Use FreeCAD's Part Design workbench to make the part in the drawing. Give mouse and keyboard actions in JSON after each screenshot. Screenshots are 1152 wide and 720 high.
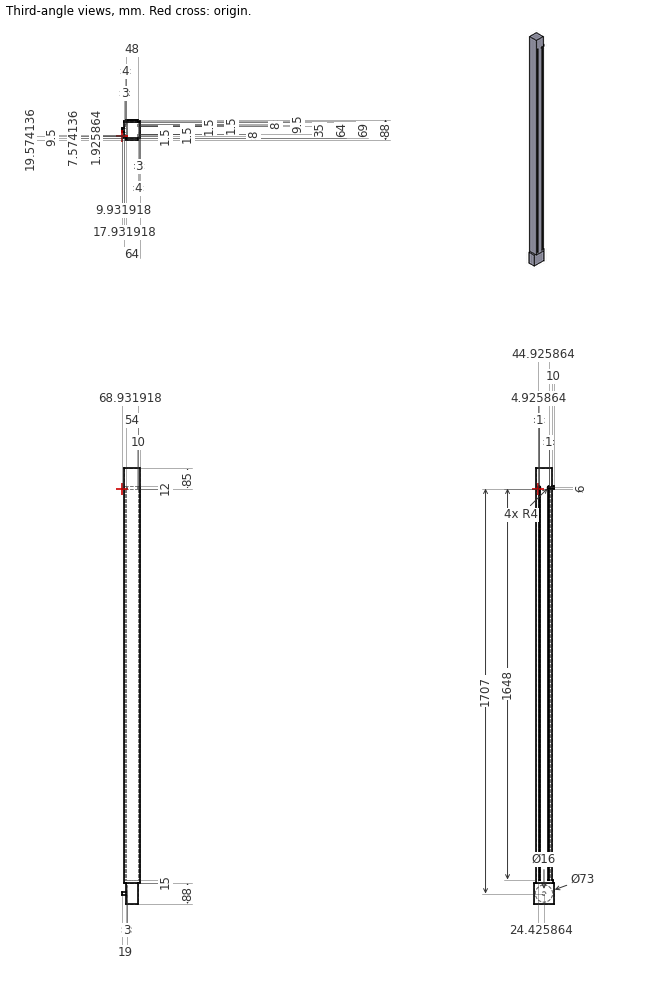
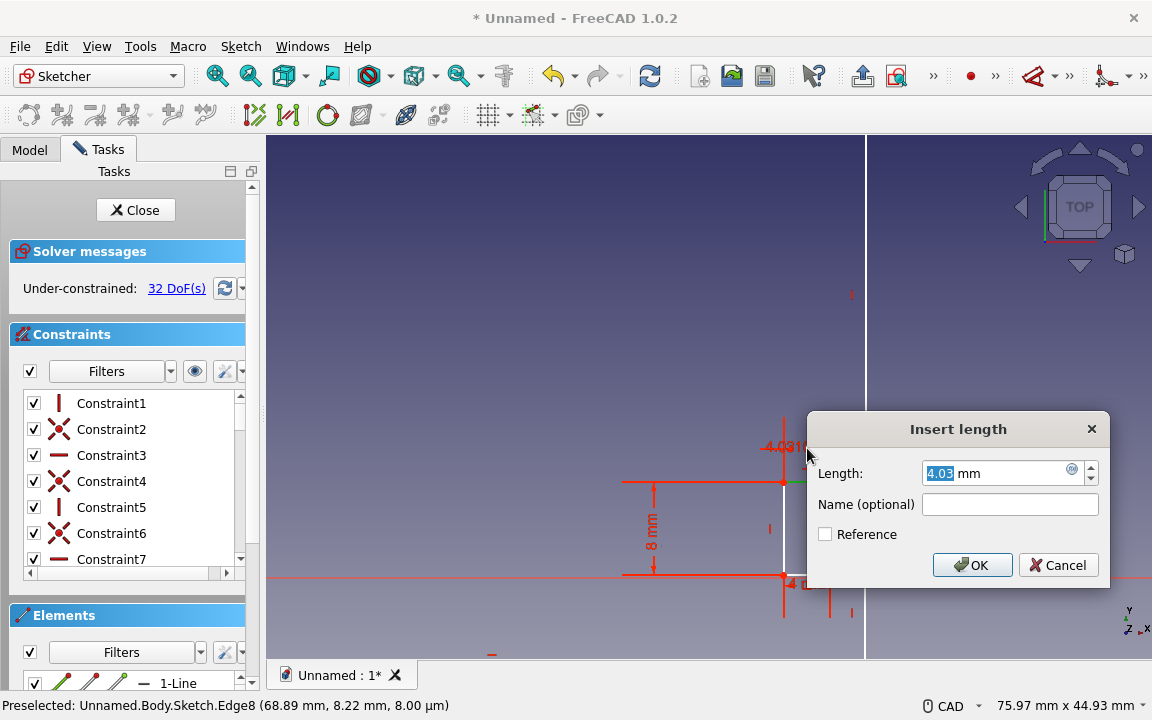
{"action": "type", "text": "4"}
{"action": "key", "text": "Return"}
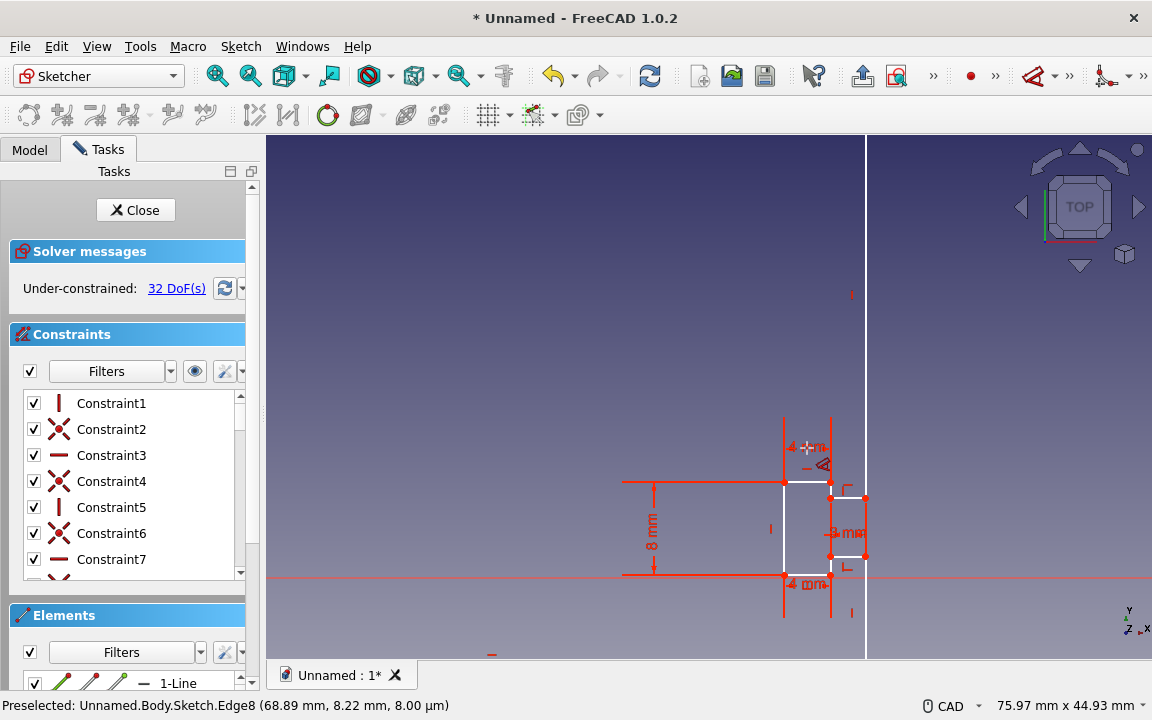
{"action": "scroll", "coordinate": [841, 498], "scroll_direction": "up", "scroll_amount": 2}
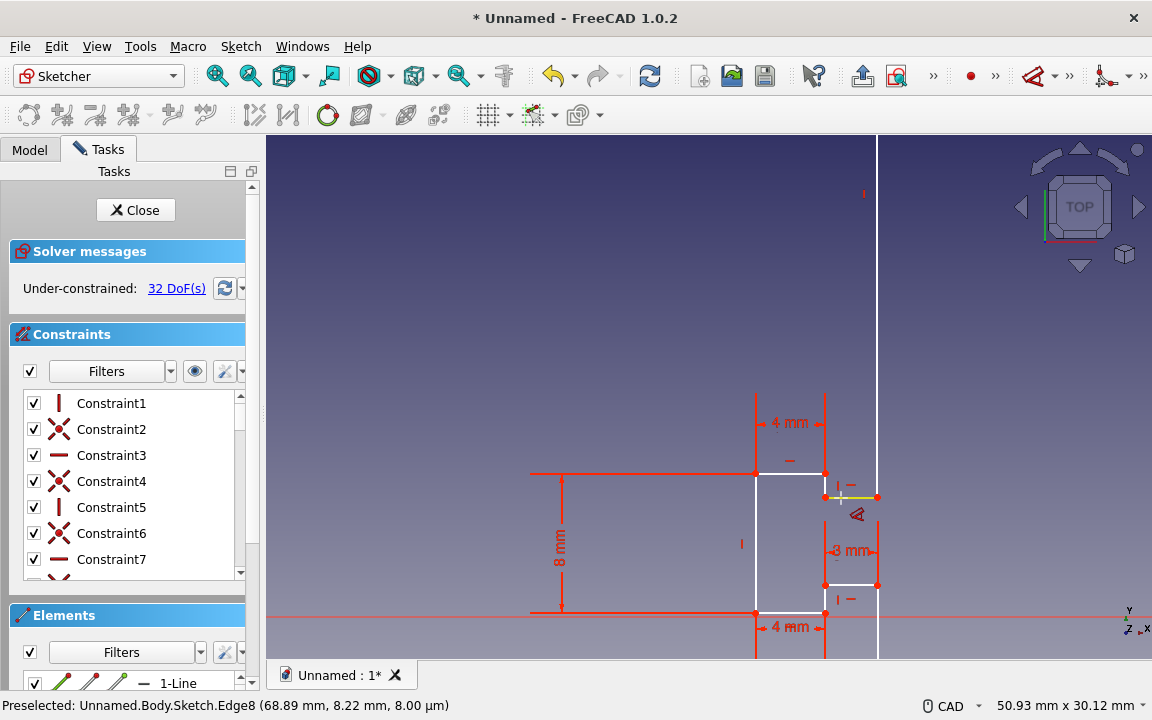
{"action": "left_click", "coordinate": [841, 498]}
{"action": "left_click", "coordinate": [851, 464]}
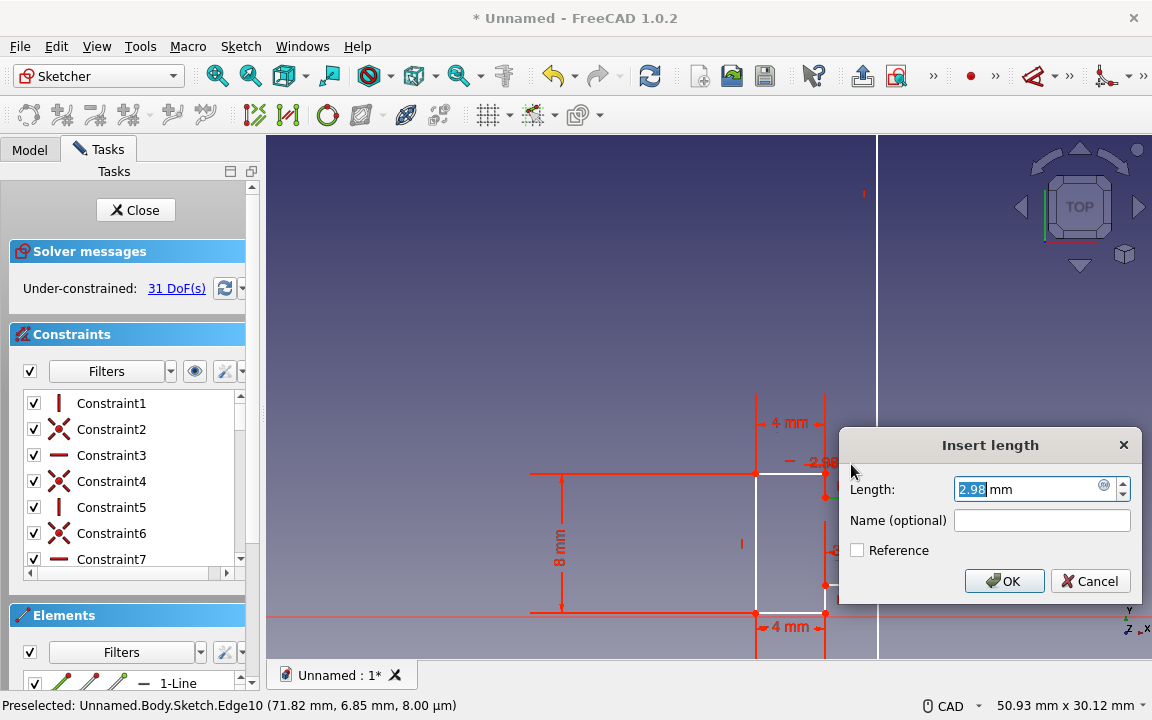
{"action": "type", "text": "3"}
{"action": "key", "text": "Return"}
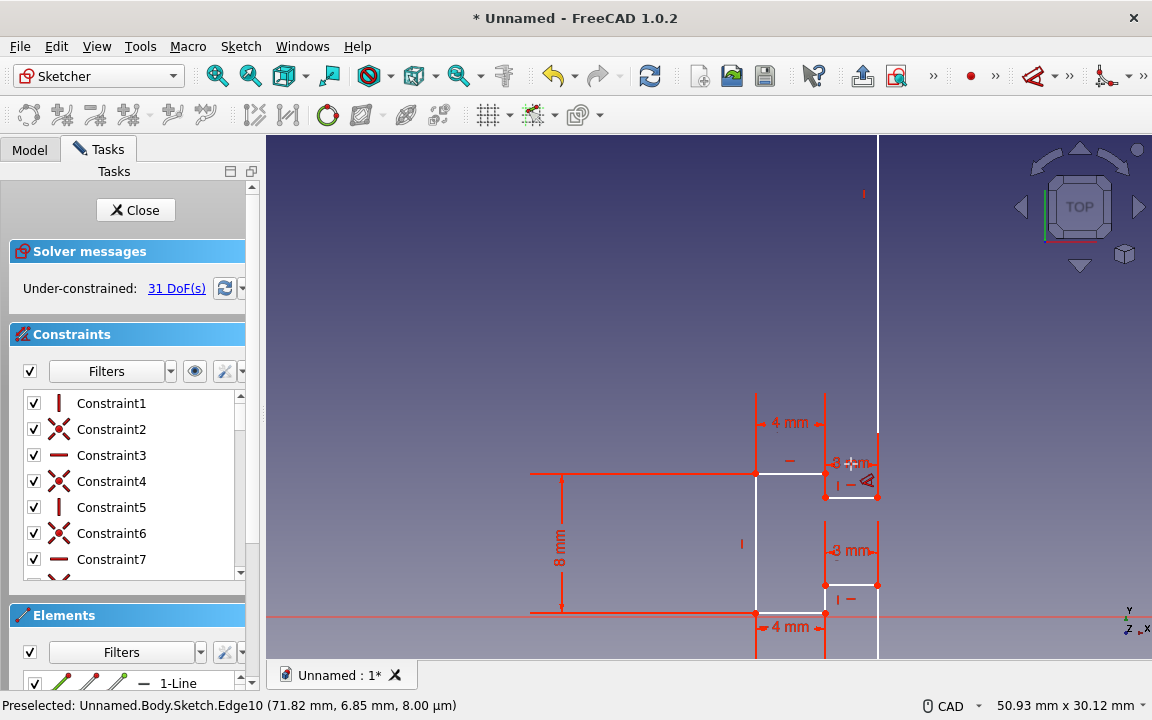
{"action": "scroll", "coordinate": [815, 485], "scroll_direction": "down", "scroll_amount": 6}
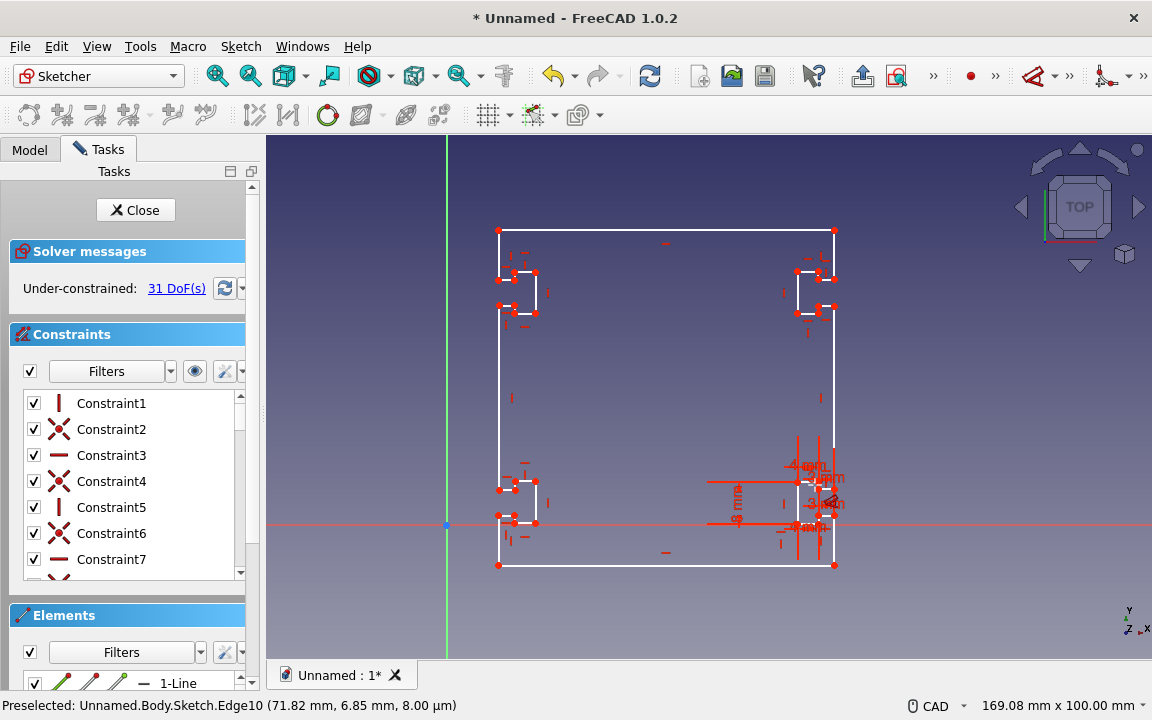
{"action": "scroll", "coordinate": [830, 306], "scroll_direction": "up", "scroll_amount": 6}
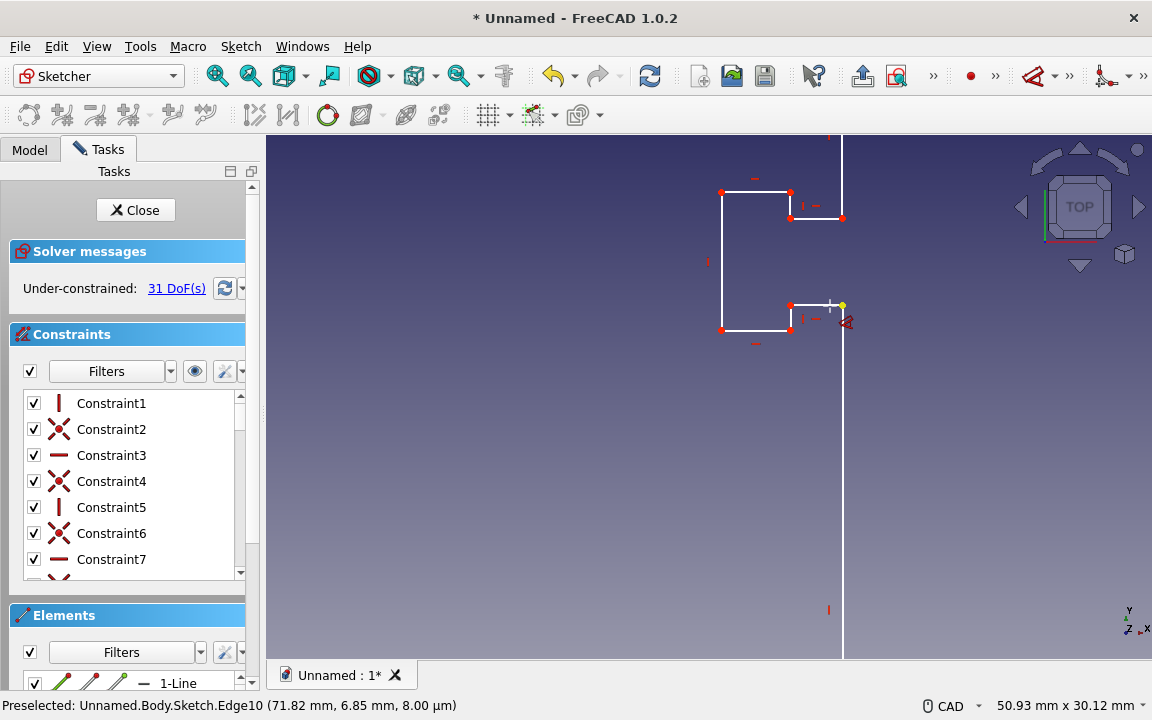
{"action": "left_click", "coordinate": [827, 305]}
{"action": "left_click", "coordinate": [817, 271]}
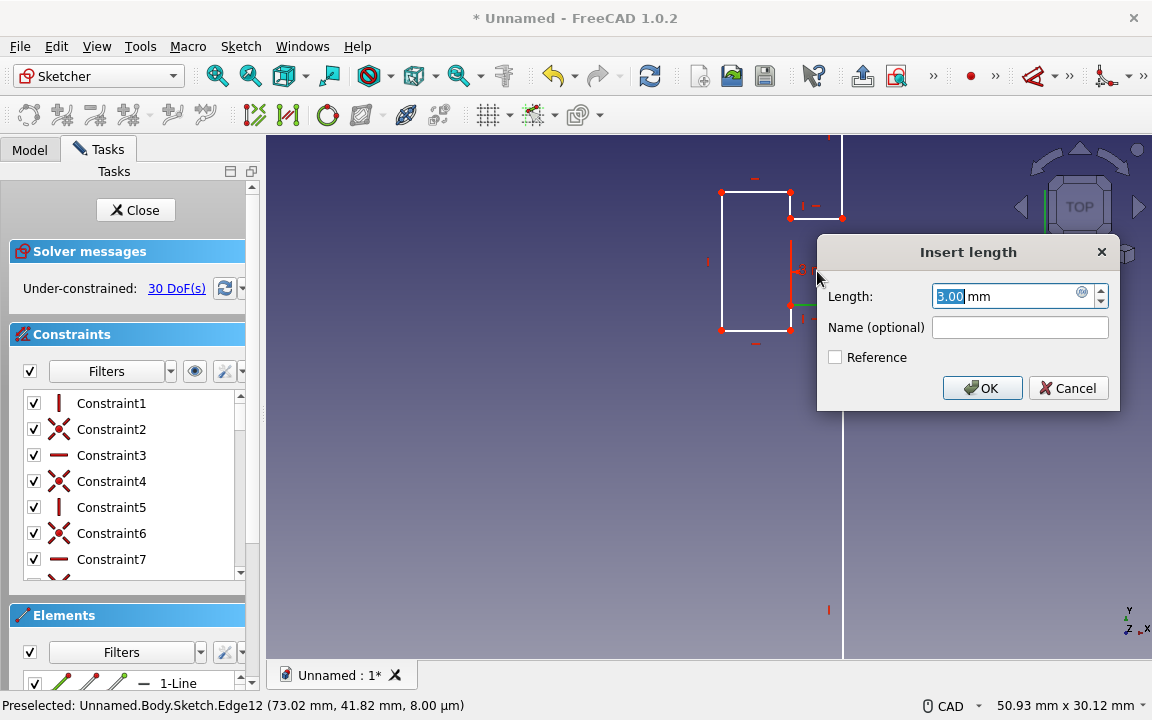
{"action": "type", "text": "3"}
{"action": "key", "text": "Return"}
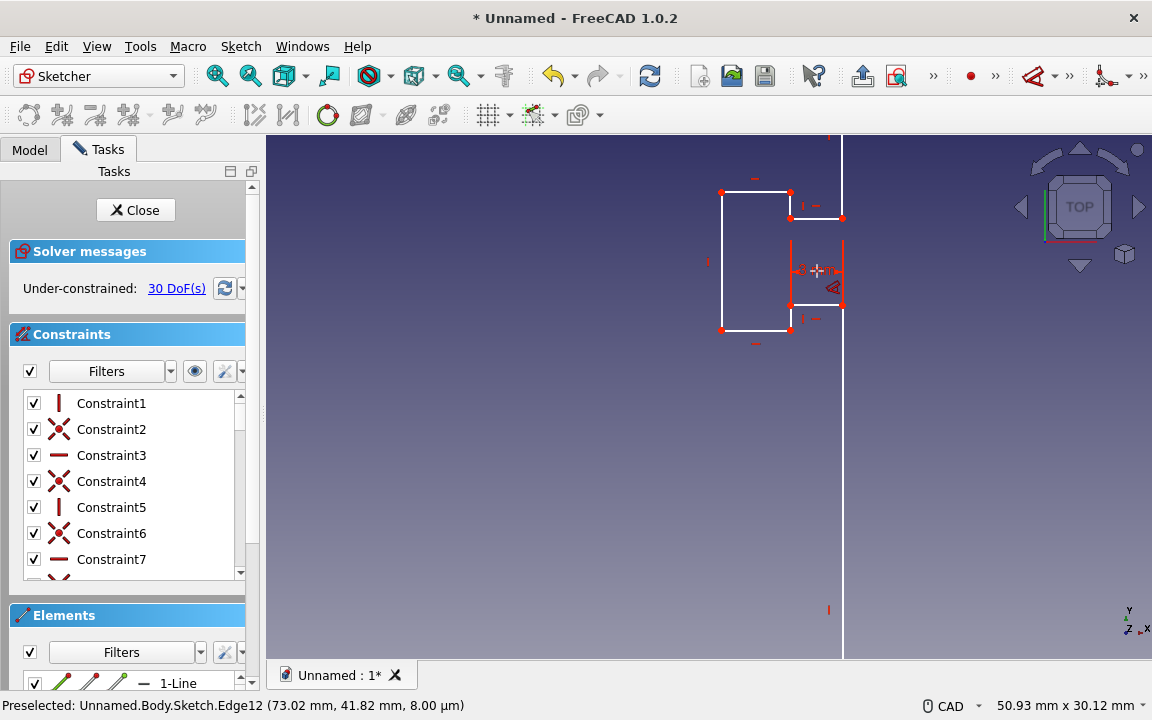
{"action": "left_click", "coordinate": [770, 331]}
{"action": "left_click", "coordinate": [756, 297]}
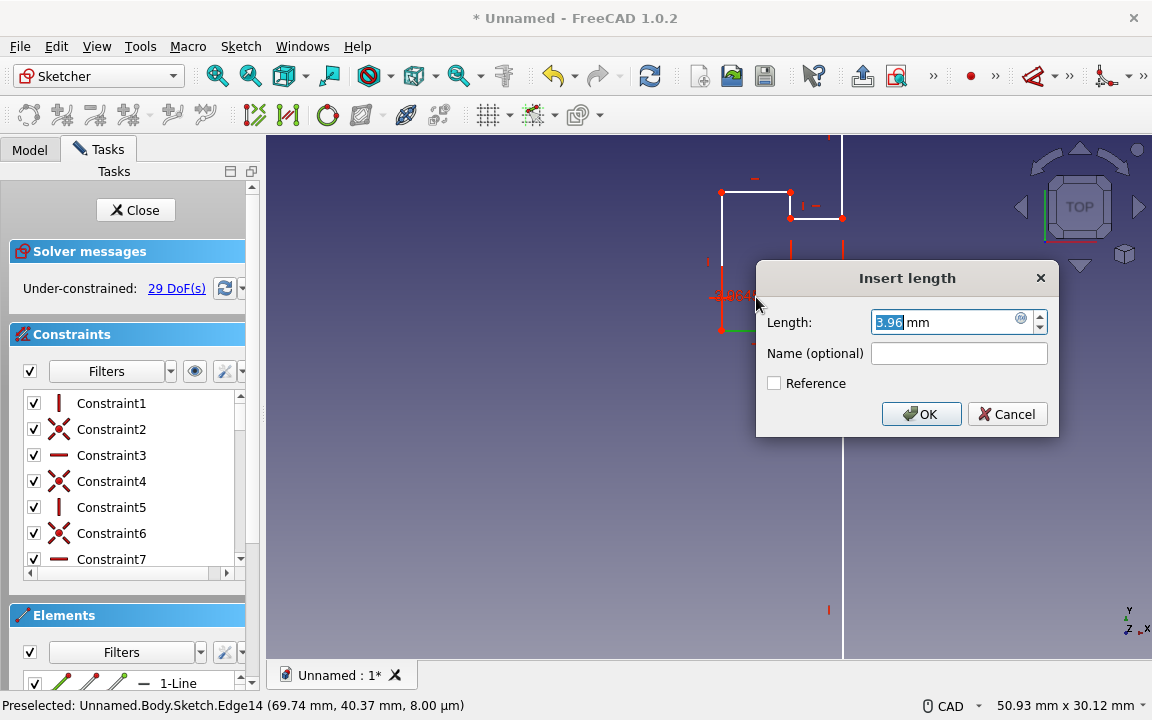
{"action": "type", "text": "4"}
{"action": "key", "text": "Return"}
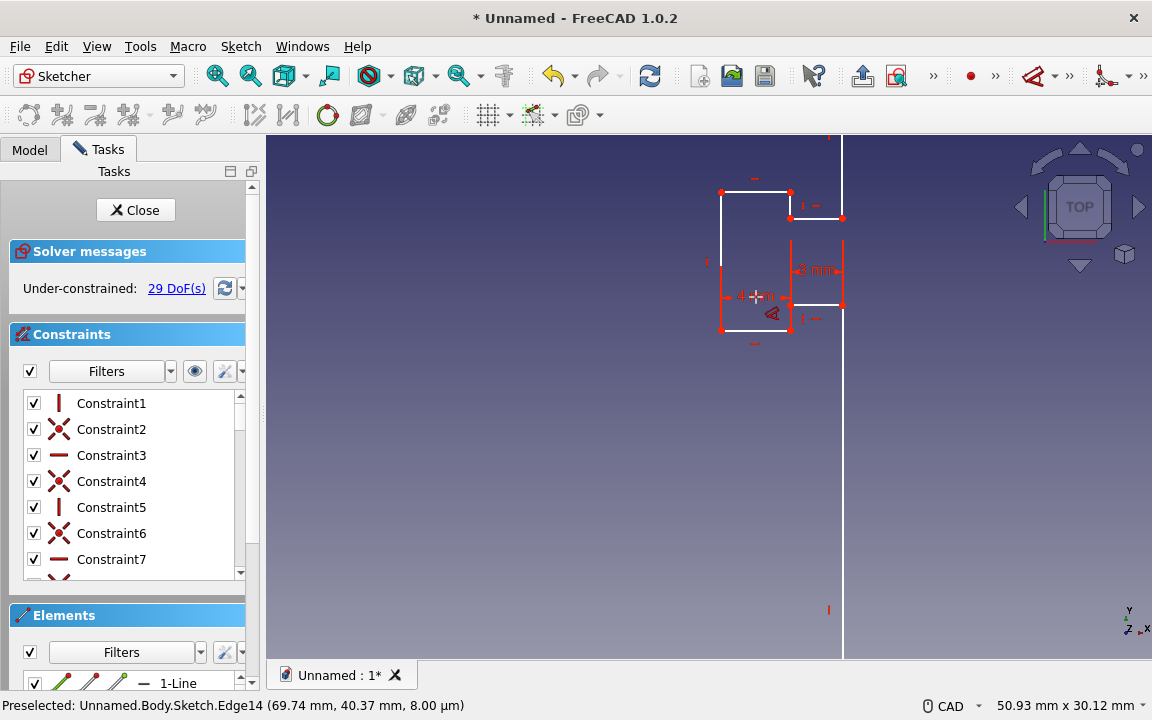
{"action": "scroll", "coordinate": [830, 306], "scroll_direction": "down", "scroll_amount": 6}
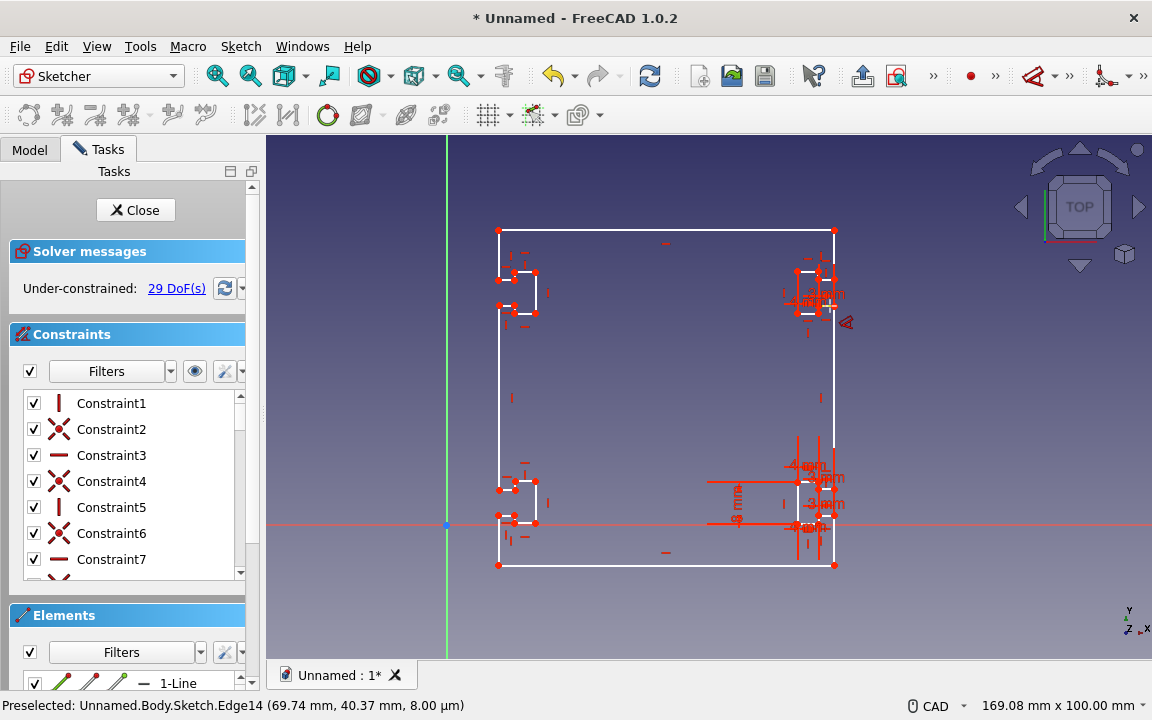
{"action": "left_click", "coordinate": [798, 301]}
{"action": "left_click", "coordinate": [740, 283]}